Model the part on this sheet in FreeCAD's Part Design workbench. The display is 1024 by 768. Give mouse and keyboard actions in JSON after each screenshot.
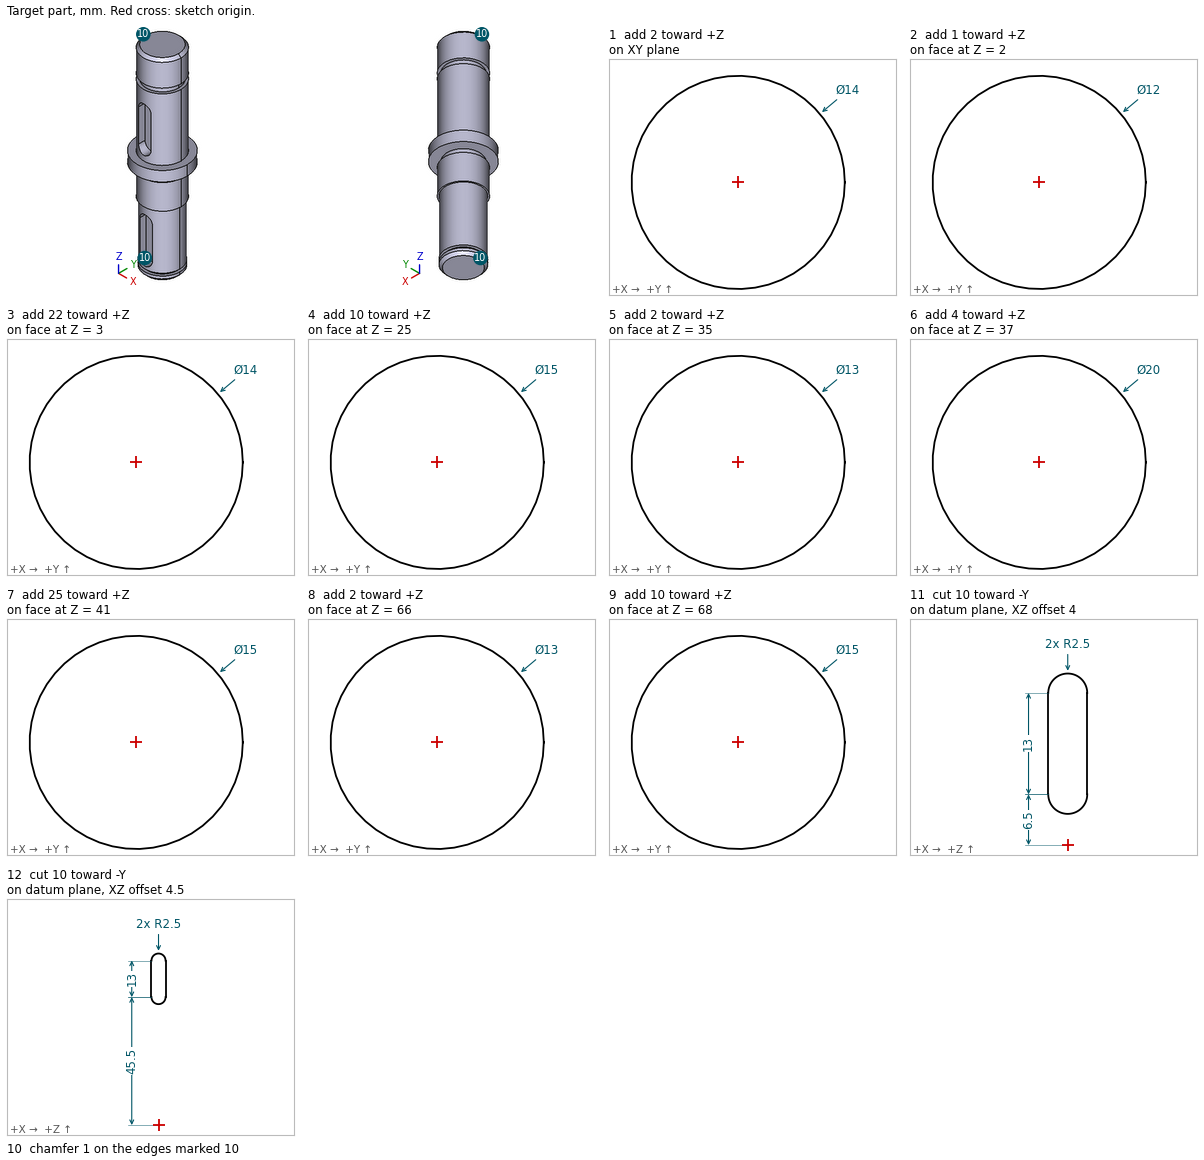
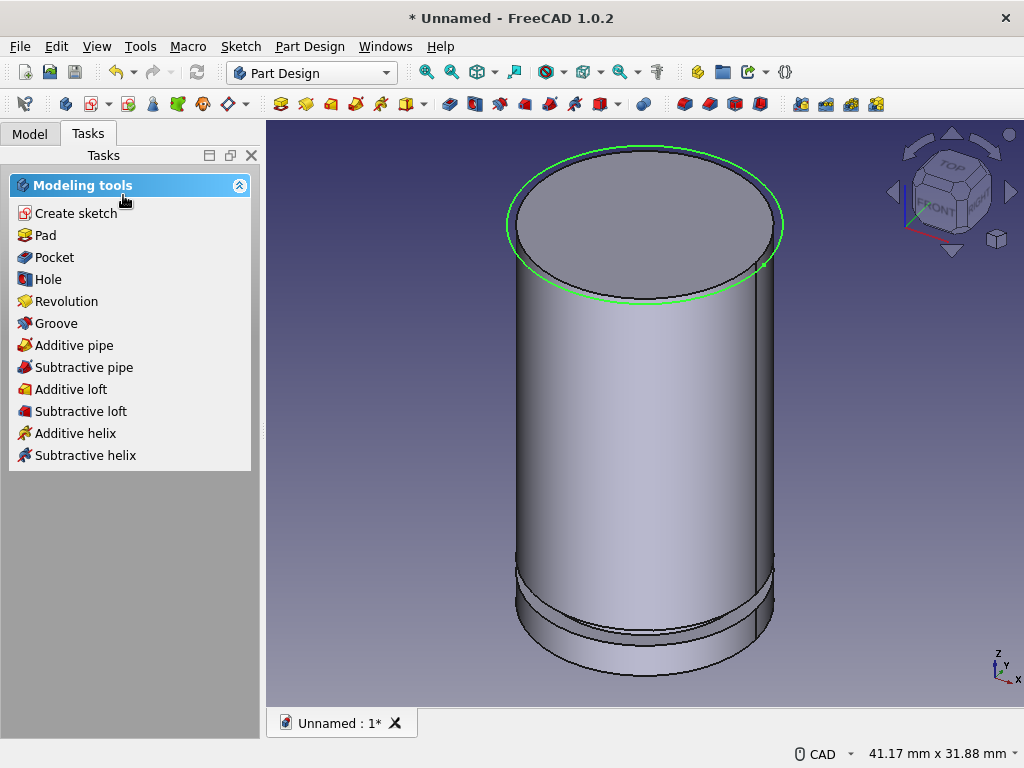
{"action": "left_click", "coordinate": [281, 104]}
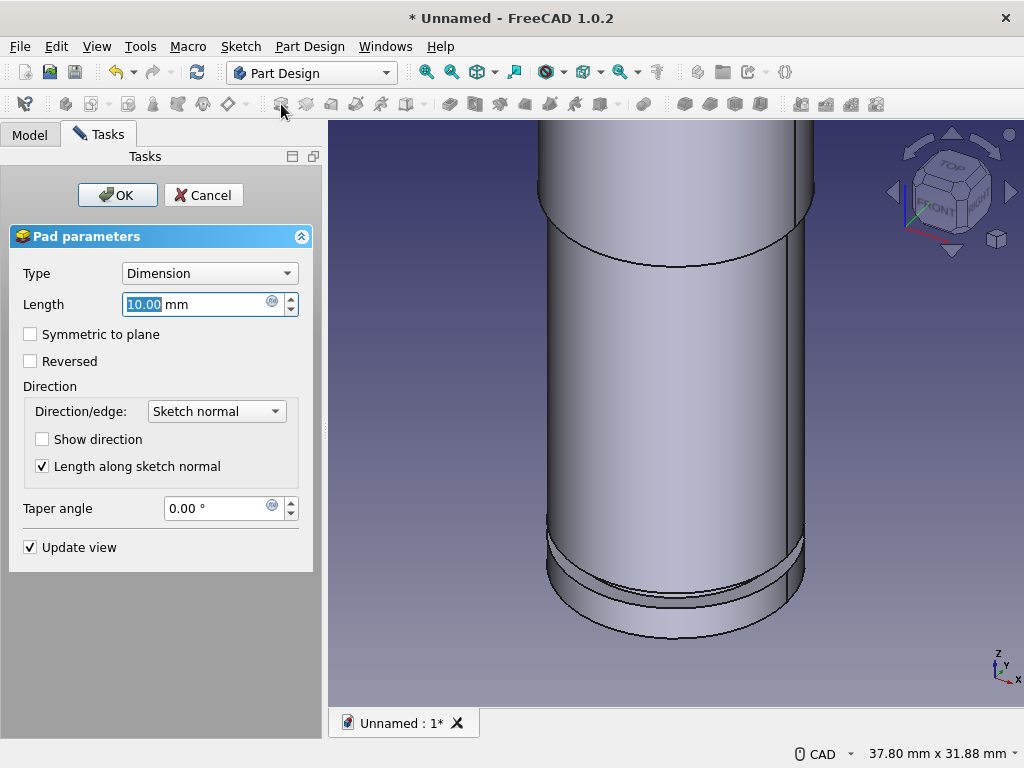
{"action": "type", "text": "10"}
{"action": "key", "text": "Tab"}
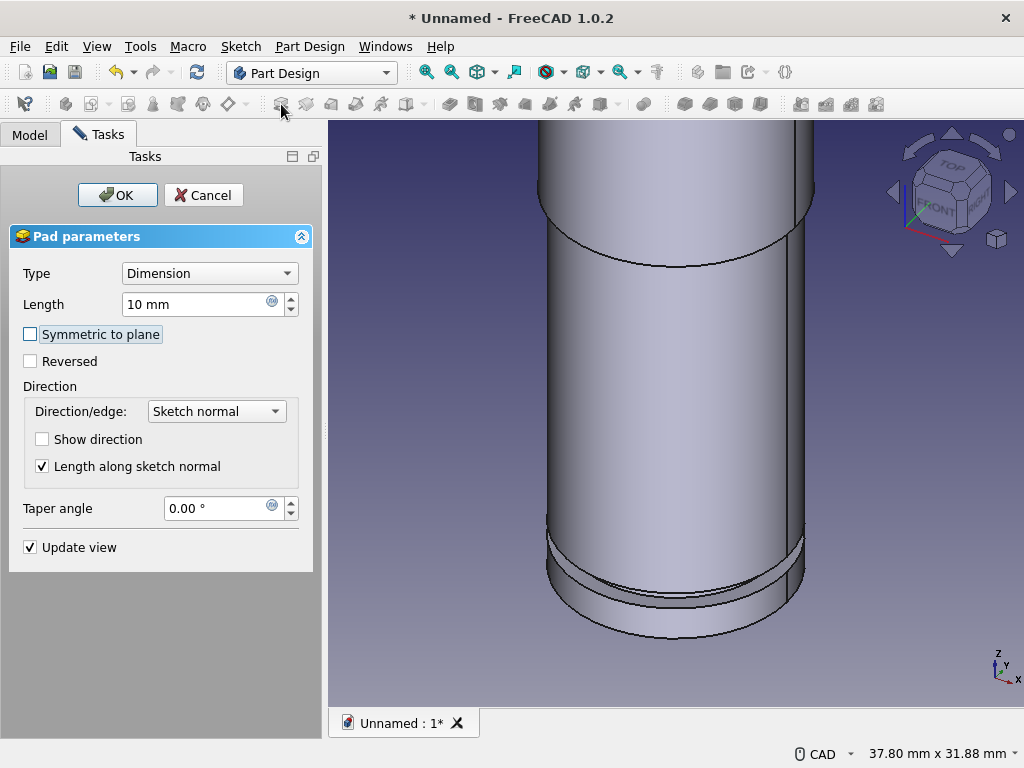
{"action": "left_click", "coordinate": [118, 195]}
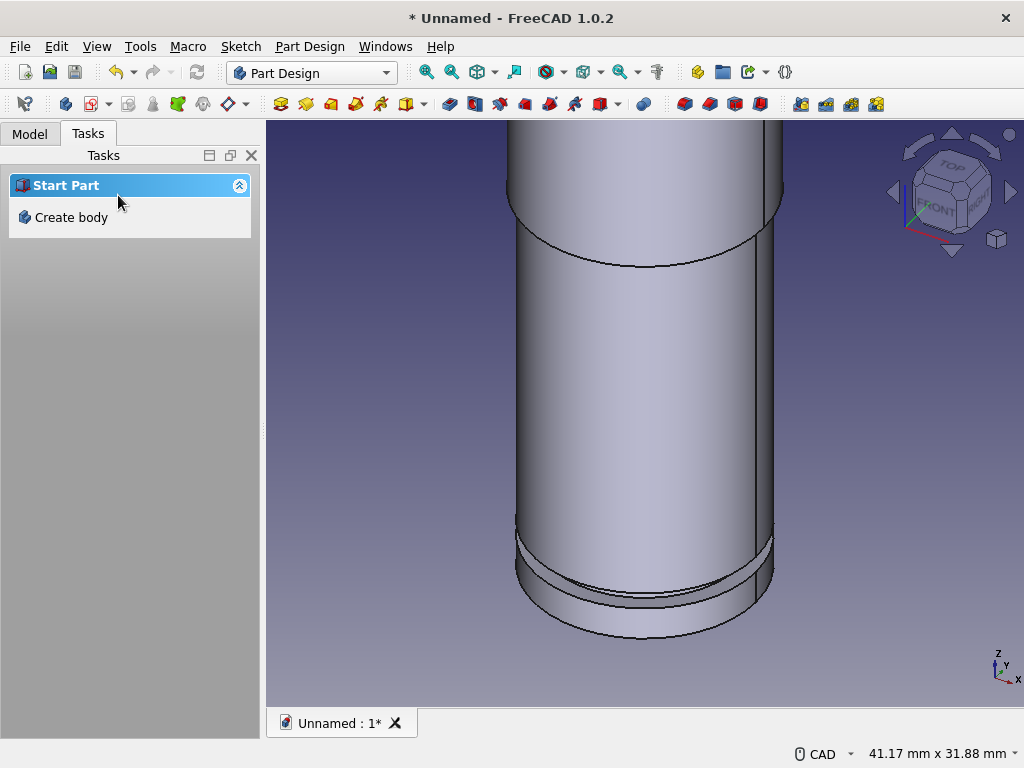
{"action": "left_click", "coordinate": [427, 72]}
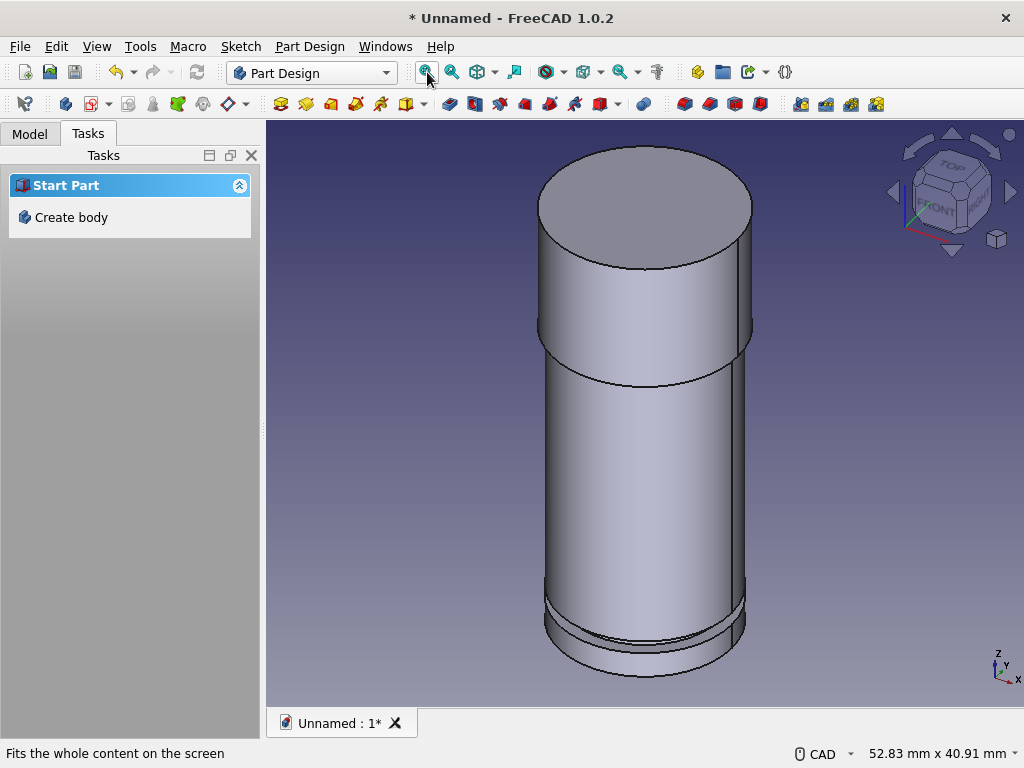
{"action": "left_click", "coordinate": [645, 207]}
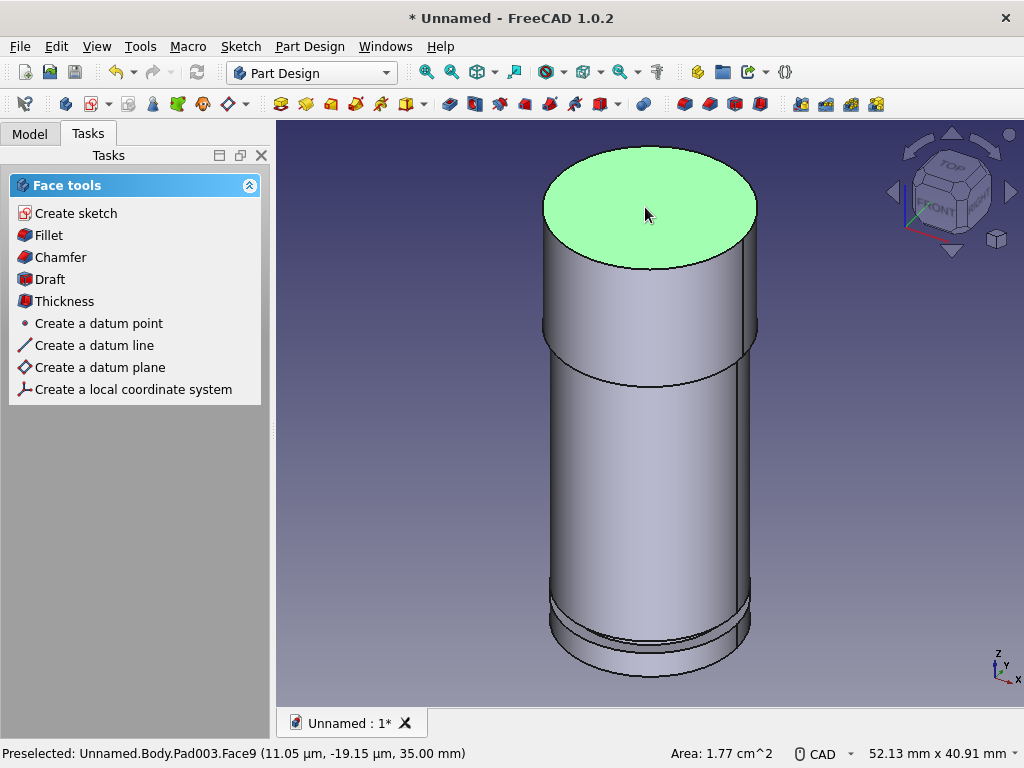
{"action": "left_click", "coordinate": [90, 104]}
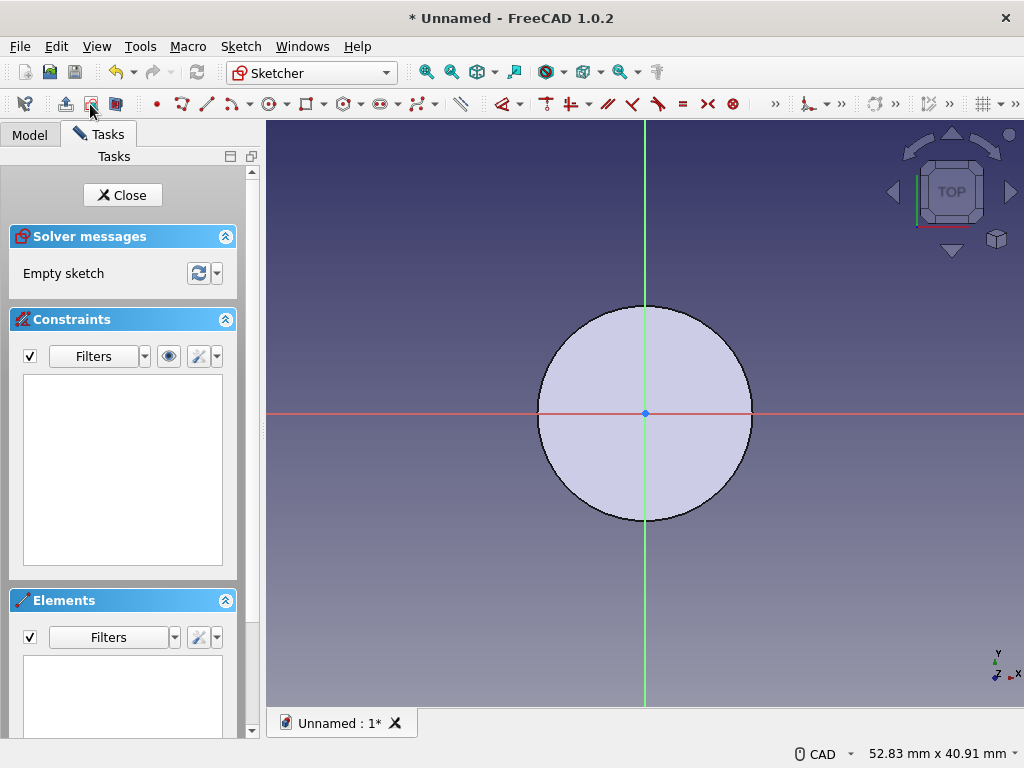
{"action": "scroll", "coordinate": [728, 414], "scroll_direction": "up", "scroll_amount": 3}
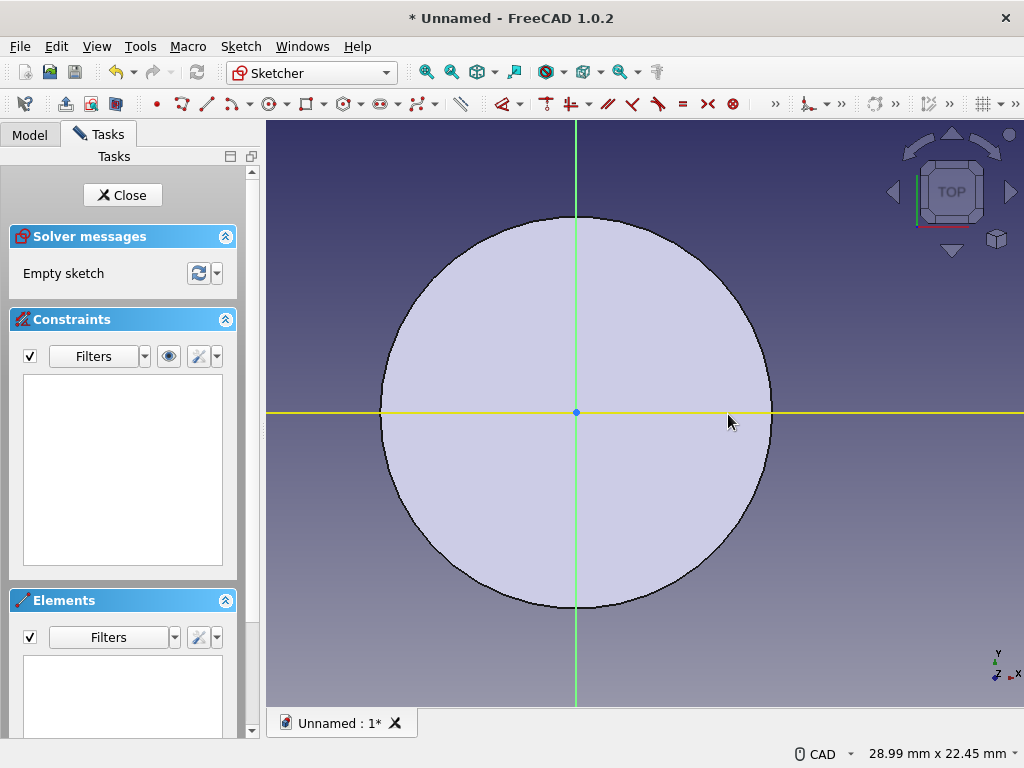
{"action": "left_click", "coordinate": [268, 104]}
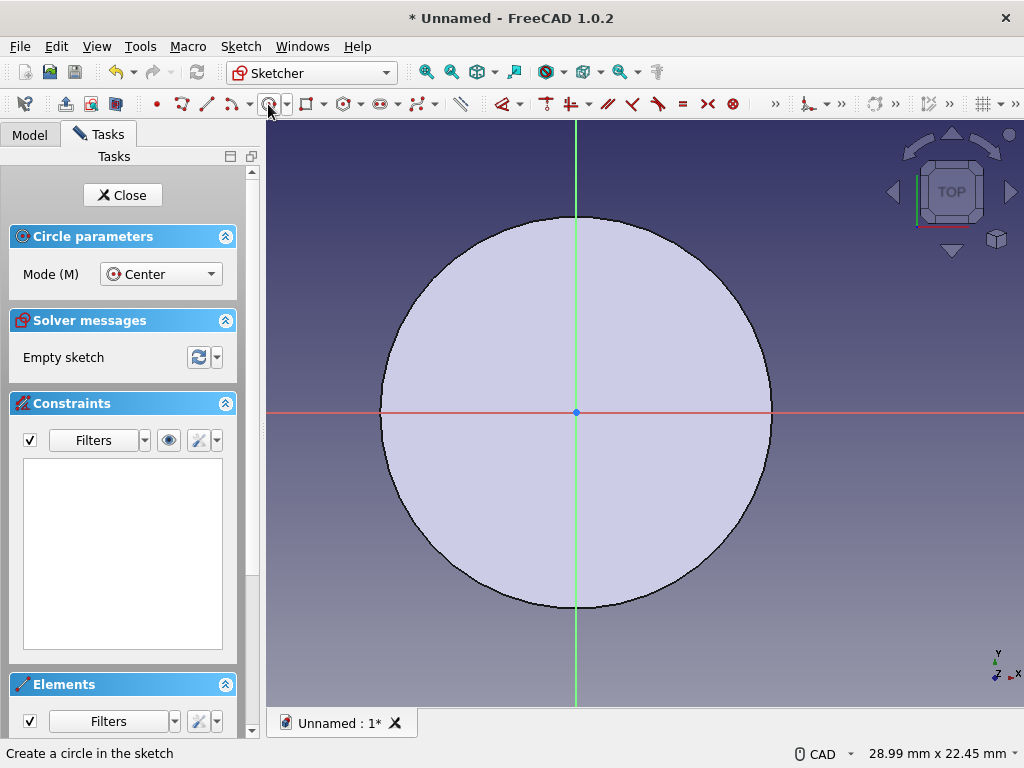
{"action": "left_click", "coordinate": [576, 413]}
{"action": "left_click", "coordinate": [696, 293]}
{"action": "key", "text": "Escape"}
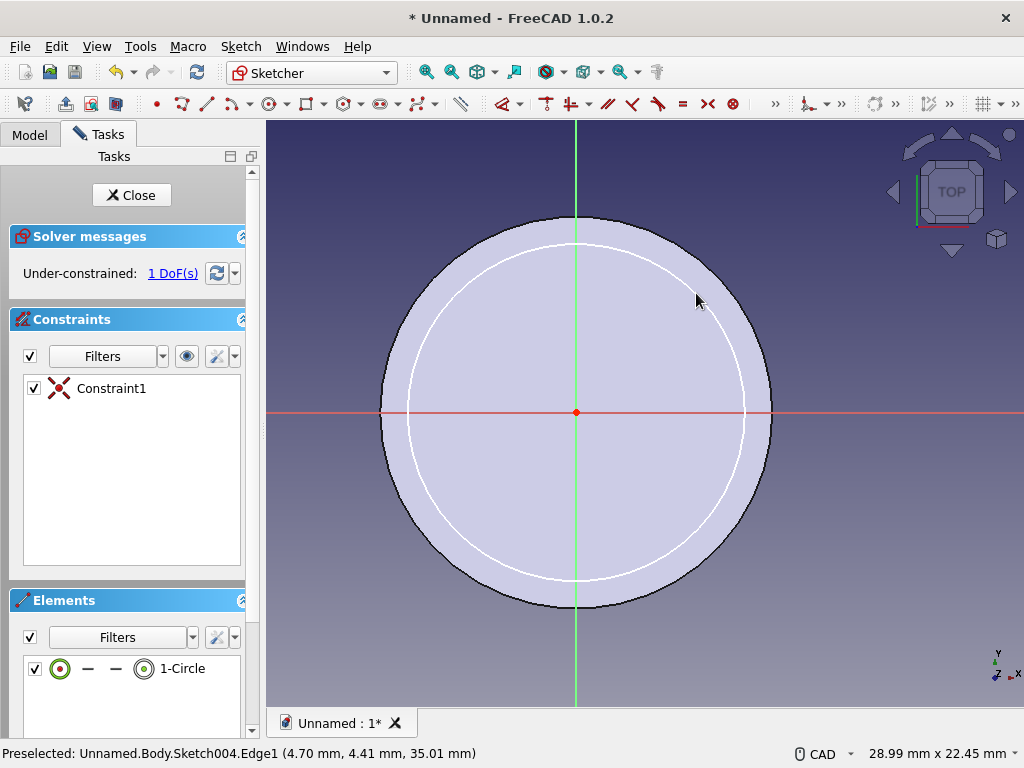
{"action": "left_click", "coordinate": [502, 104]}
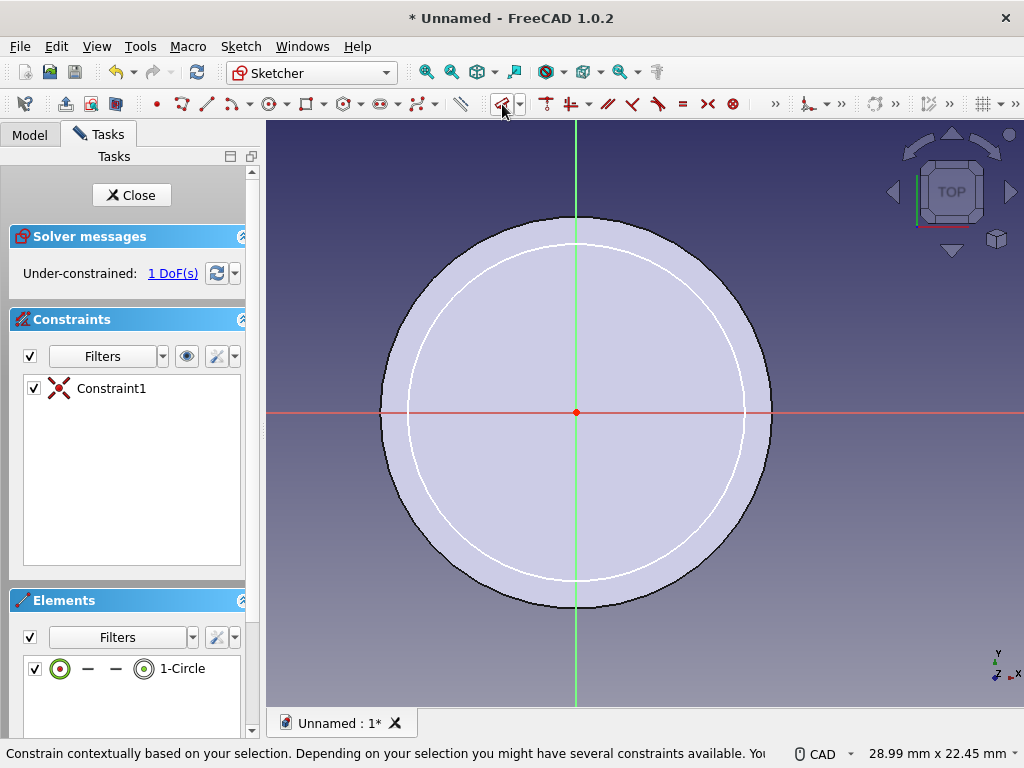
{"action": "left_click", "coordinate": [695, 293]}
{"action": "left_click", "coordinate": [718, 270]}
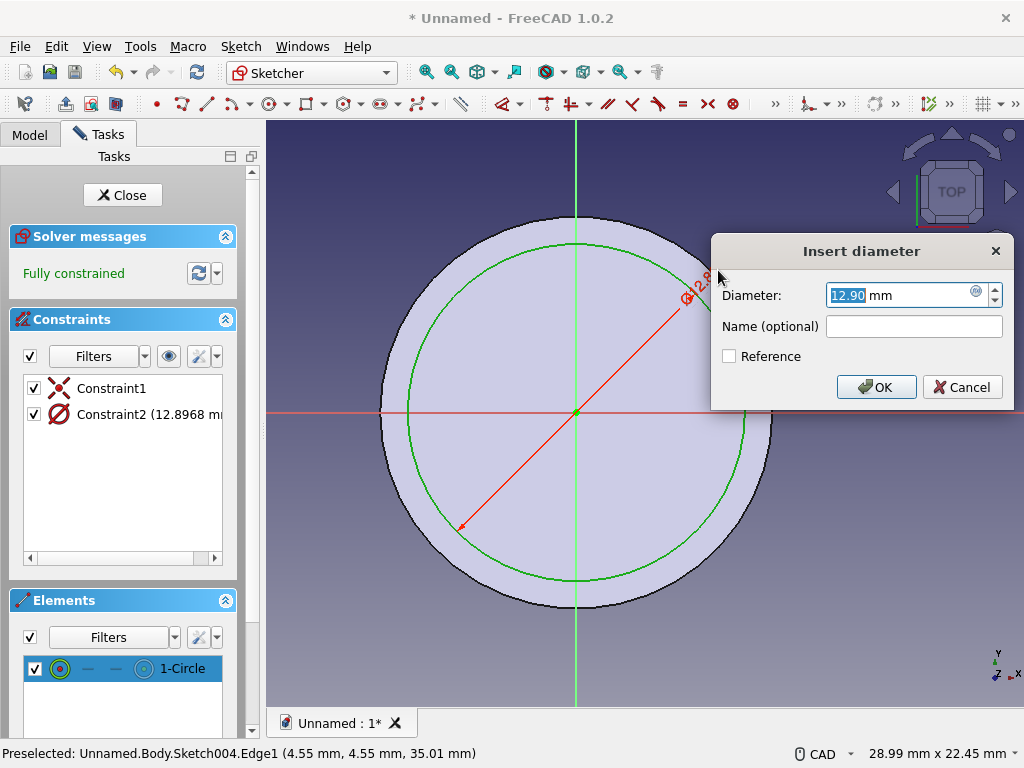
{"action": "type", "text": "13"}
{"action": "key", "text": "Return"}
{"action": "key", "text": "Escape"}